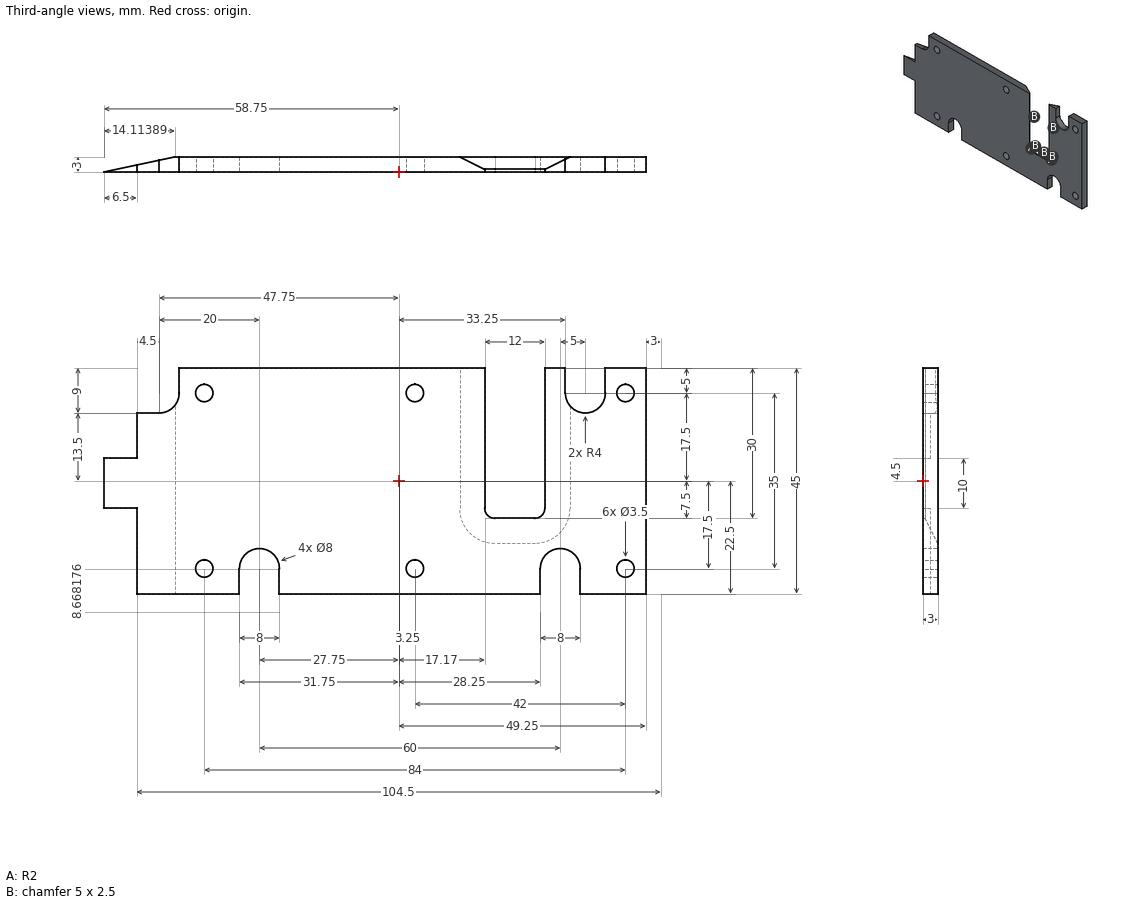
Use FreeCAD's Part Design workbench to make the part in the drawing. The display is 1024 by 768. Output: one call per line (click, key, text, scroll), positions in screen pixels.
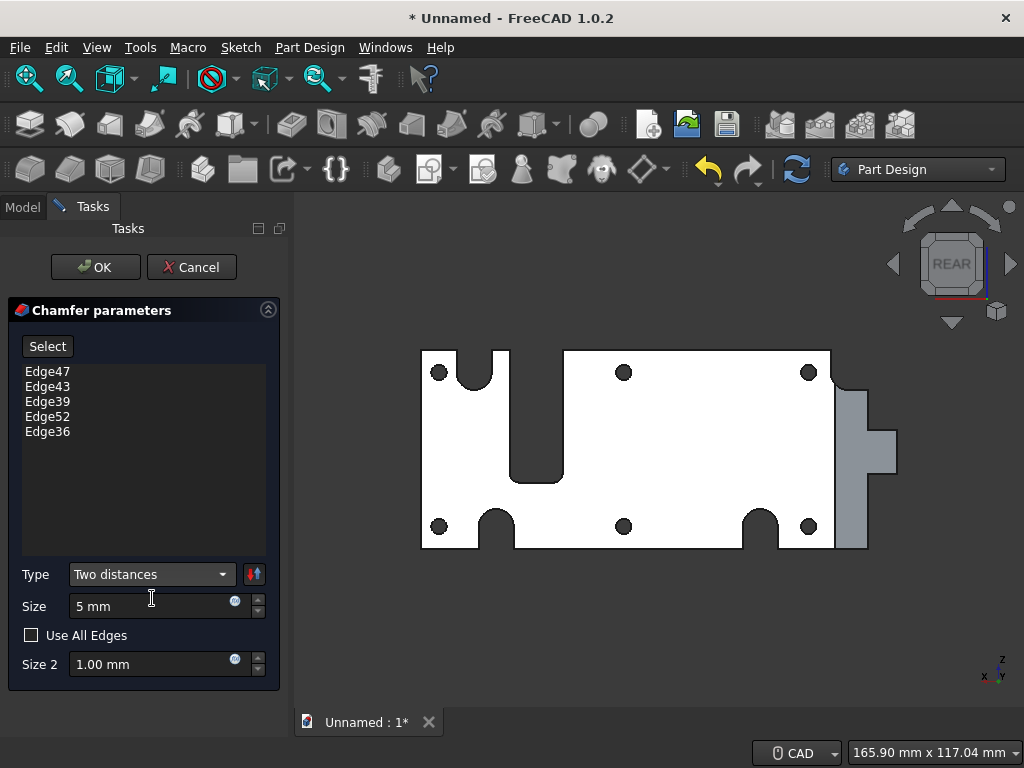
triple_click(160, 664)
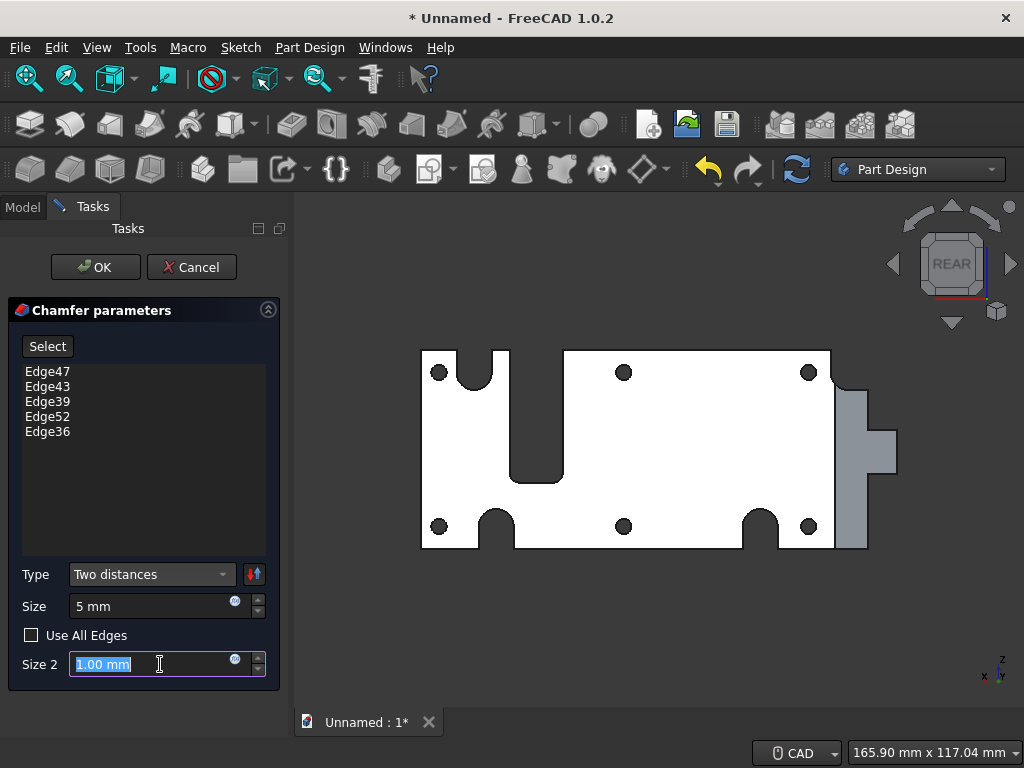
text(2.5)
key(Tab)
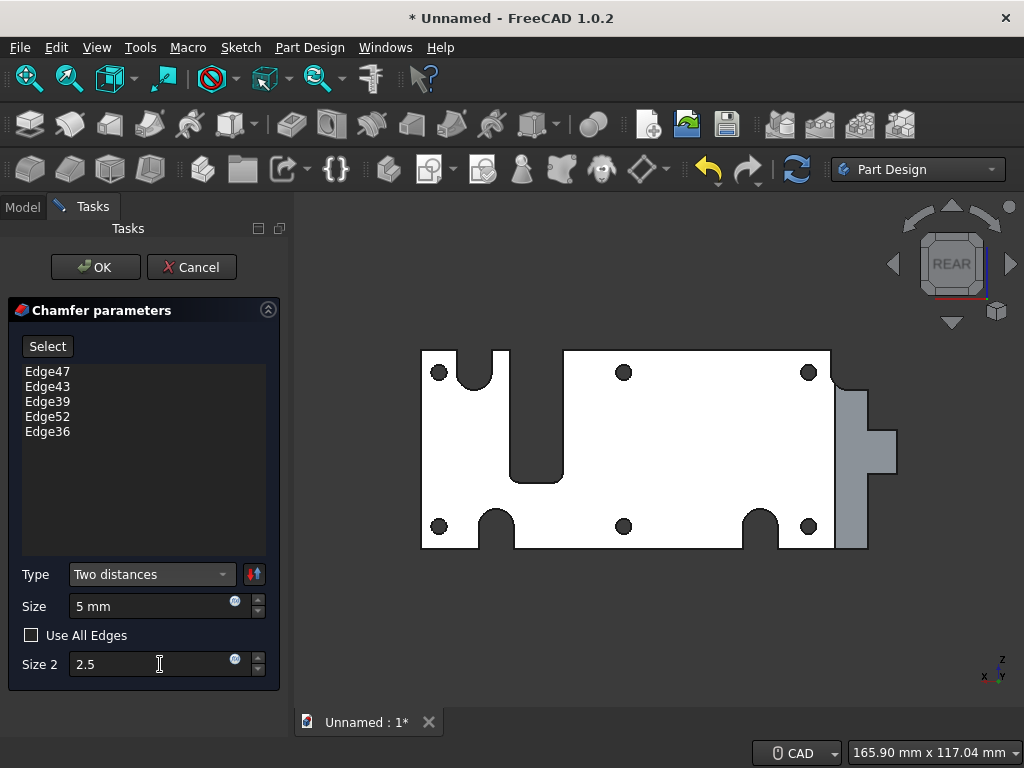
click(254, 574)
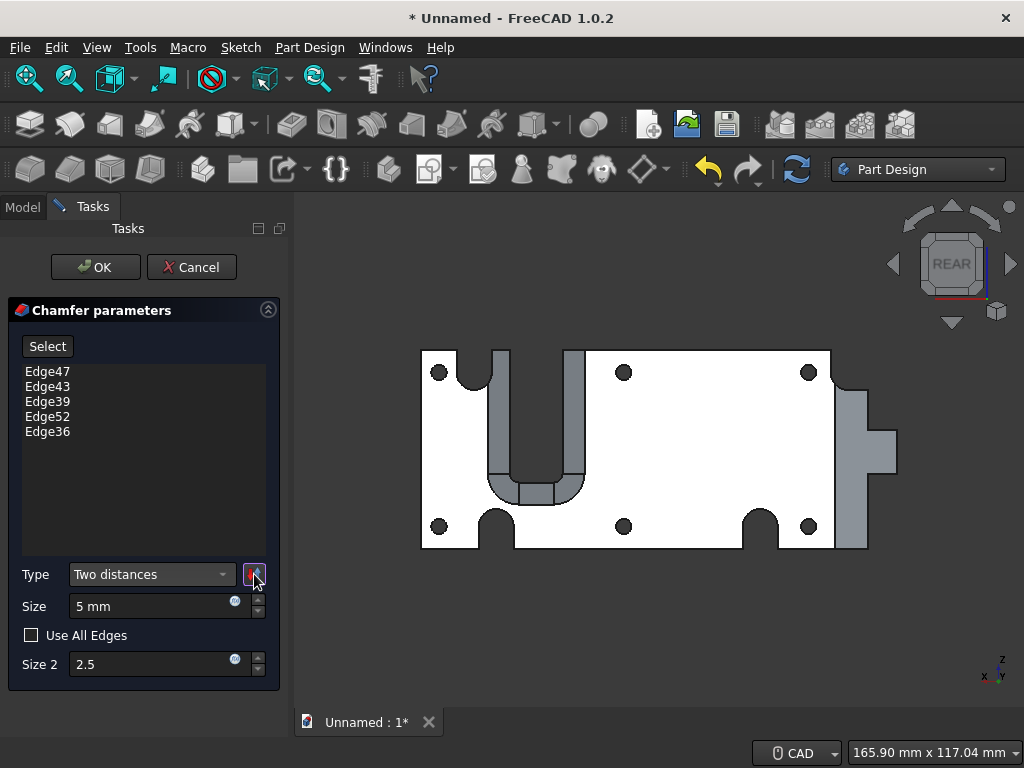
click(96, 267)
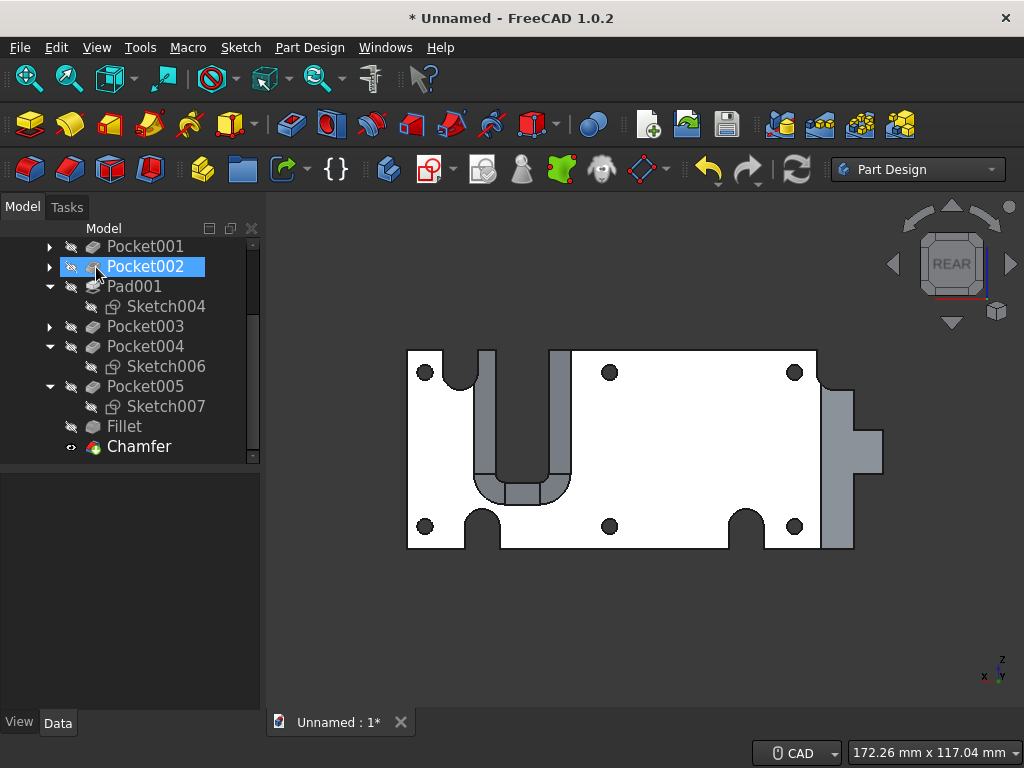
key(0)